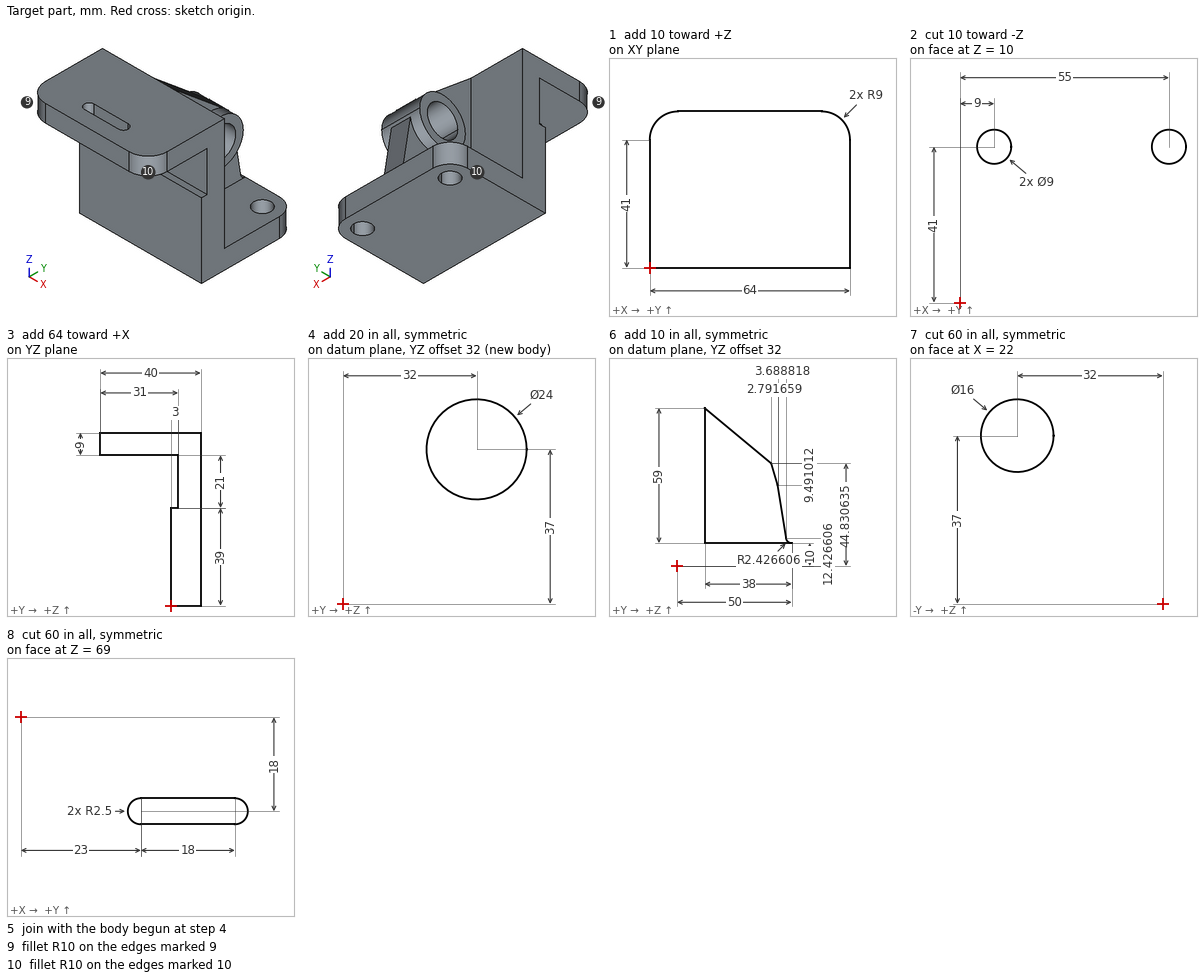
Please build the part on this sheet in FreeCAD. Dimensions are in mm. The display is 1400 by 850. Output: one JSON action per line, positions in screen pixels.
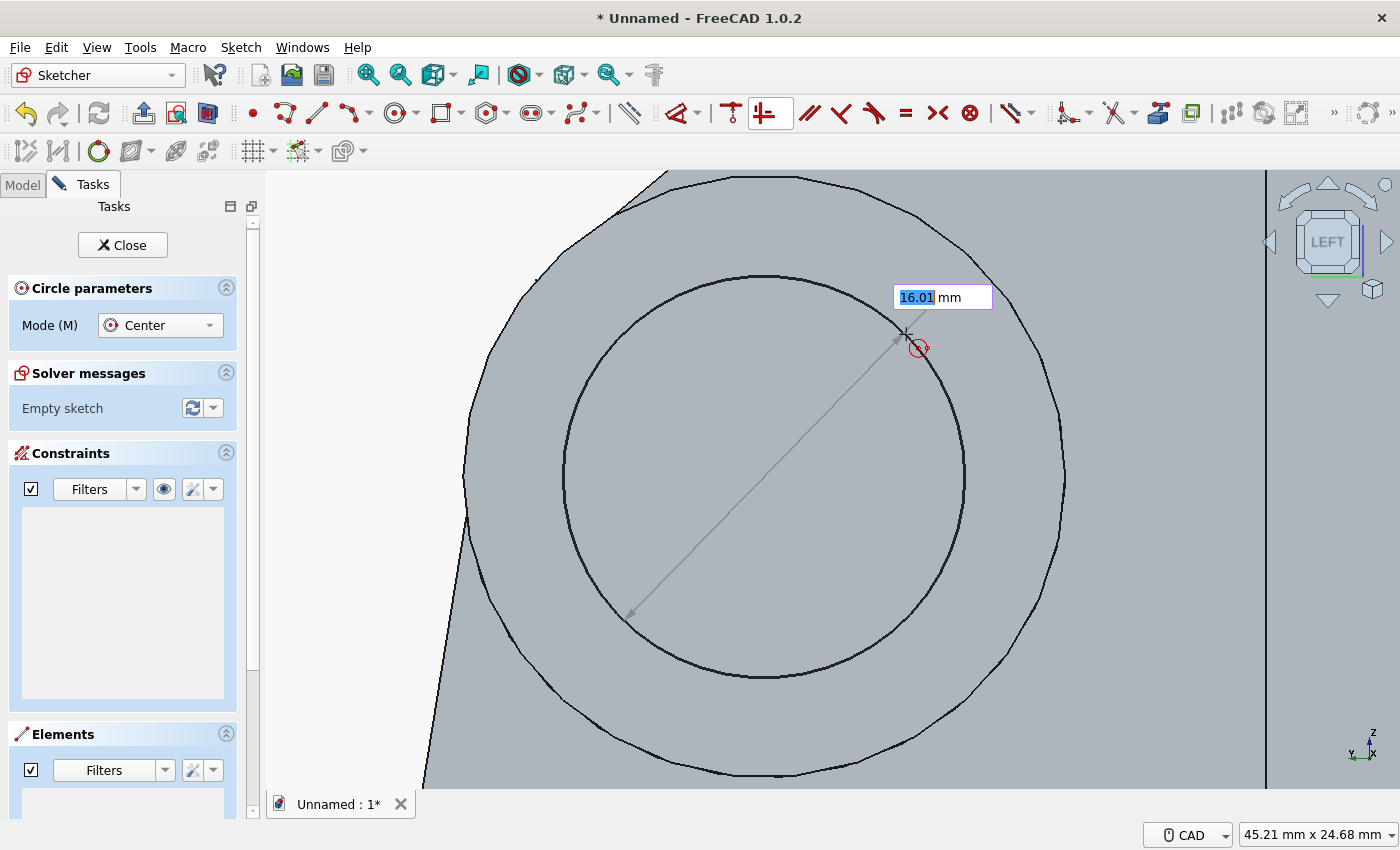
{"action": "type", "text": "16"}
{"action": "key", "text": "Return"}
{"action": "key", "text": "Escape"}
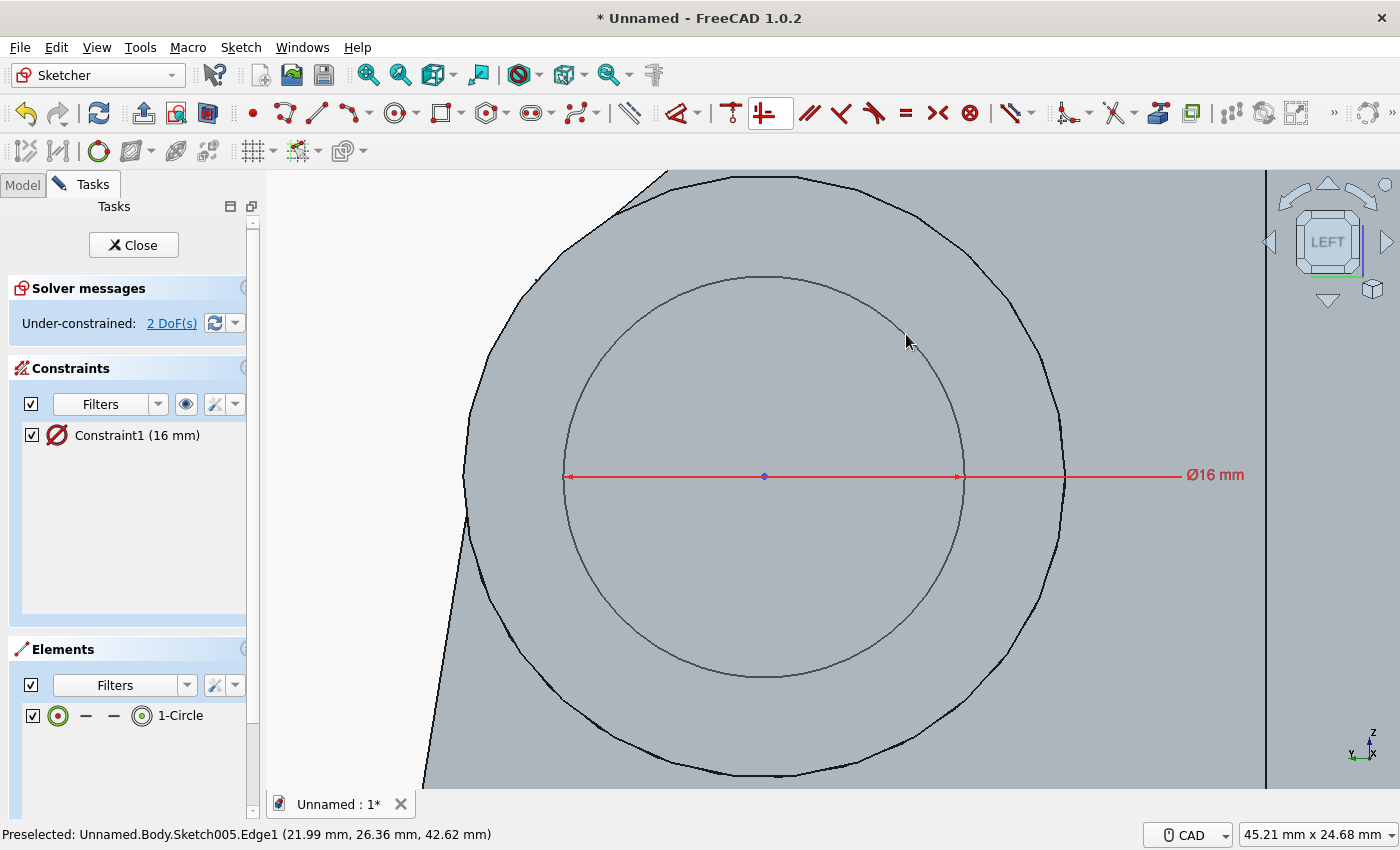
{"action": "left_click", "coordinate": [676, 114]}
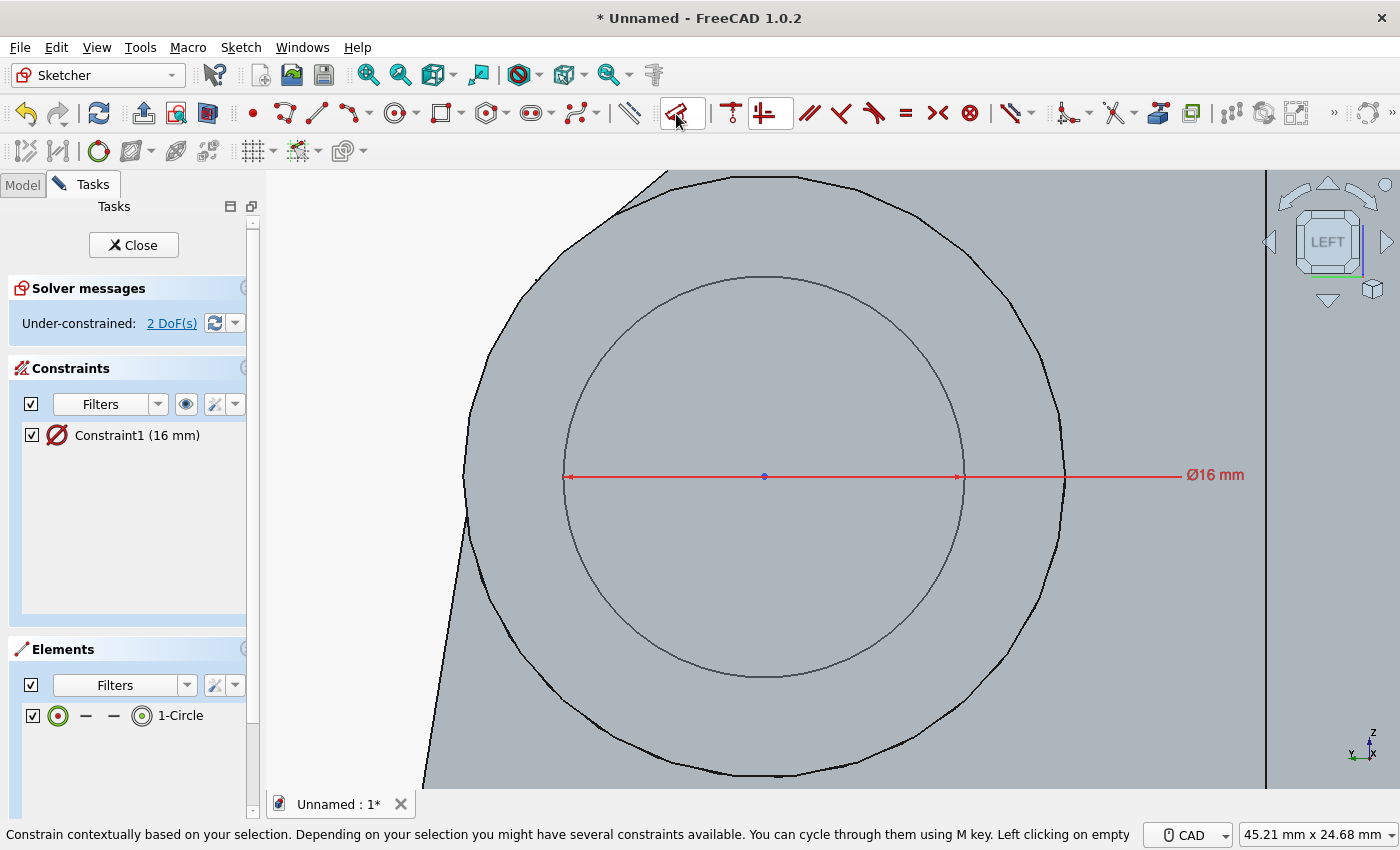
{"action": "left_click", "coordinate": [764, 477]}
{"action": "left_click", "coordinate": [999, 443]}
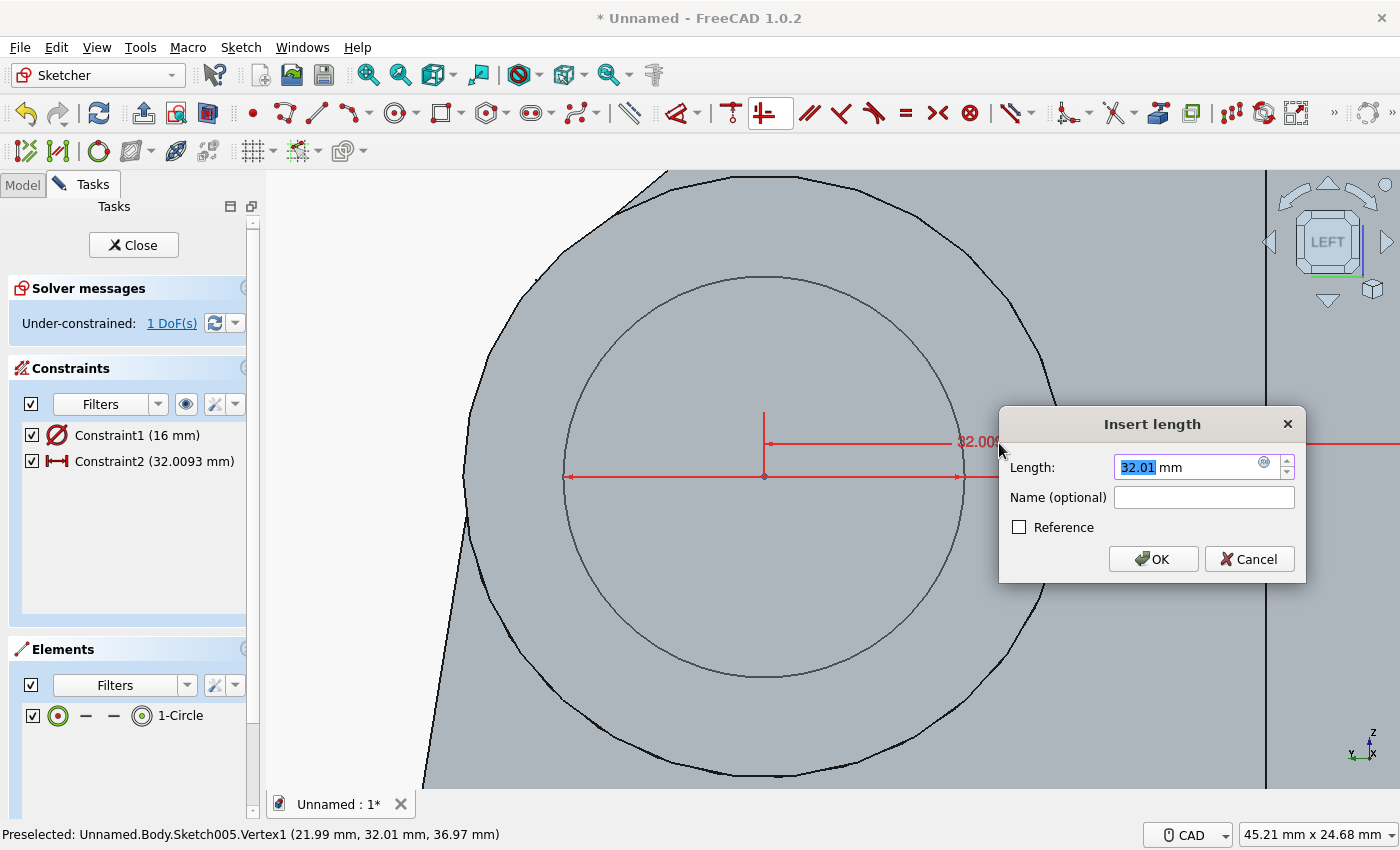
{"action": "type", "text": "32"}
{"action": "key", "text": "Return"}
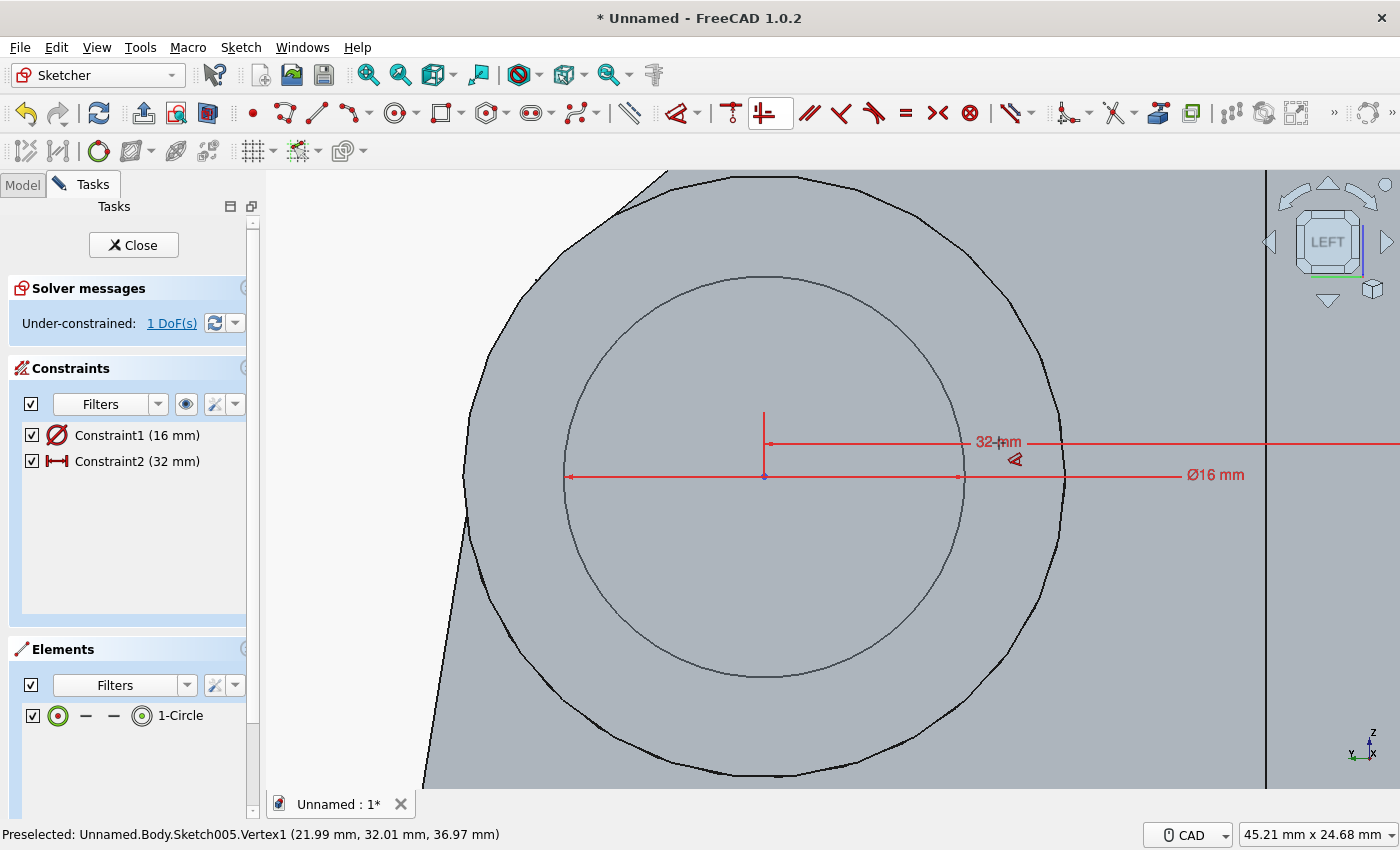
{"action": "left_click", "coordinate": [764, 477]}
{"action": "left_click", "coordinate": [730, 619]}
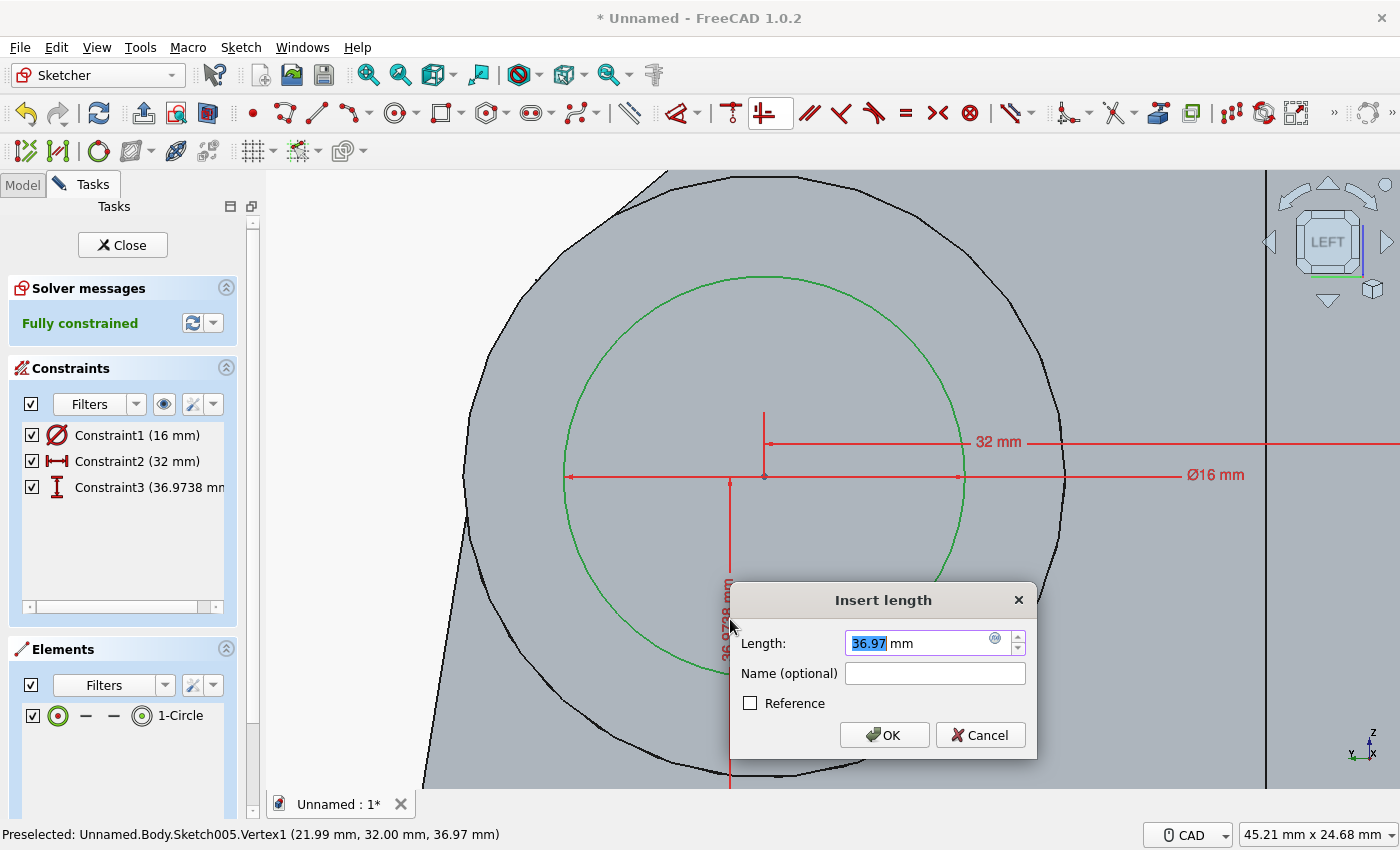
{"action": "type", "text": "37"}
{"action": "key", "text": "Return"}
{"action": "key", "text": "Escape"}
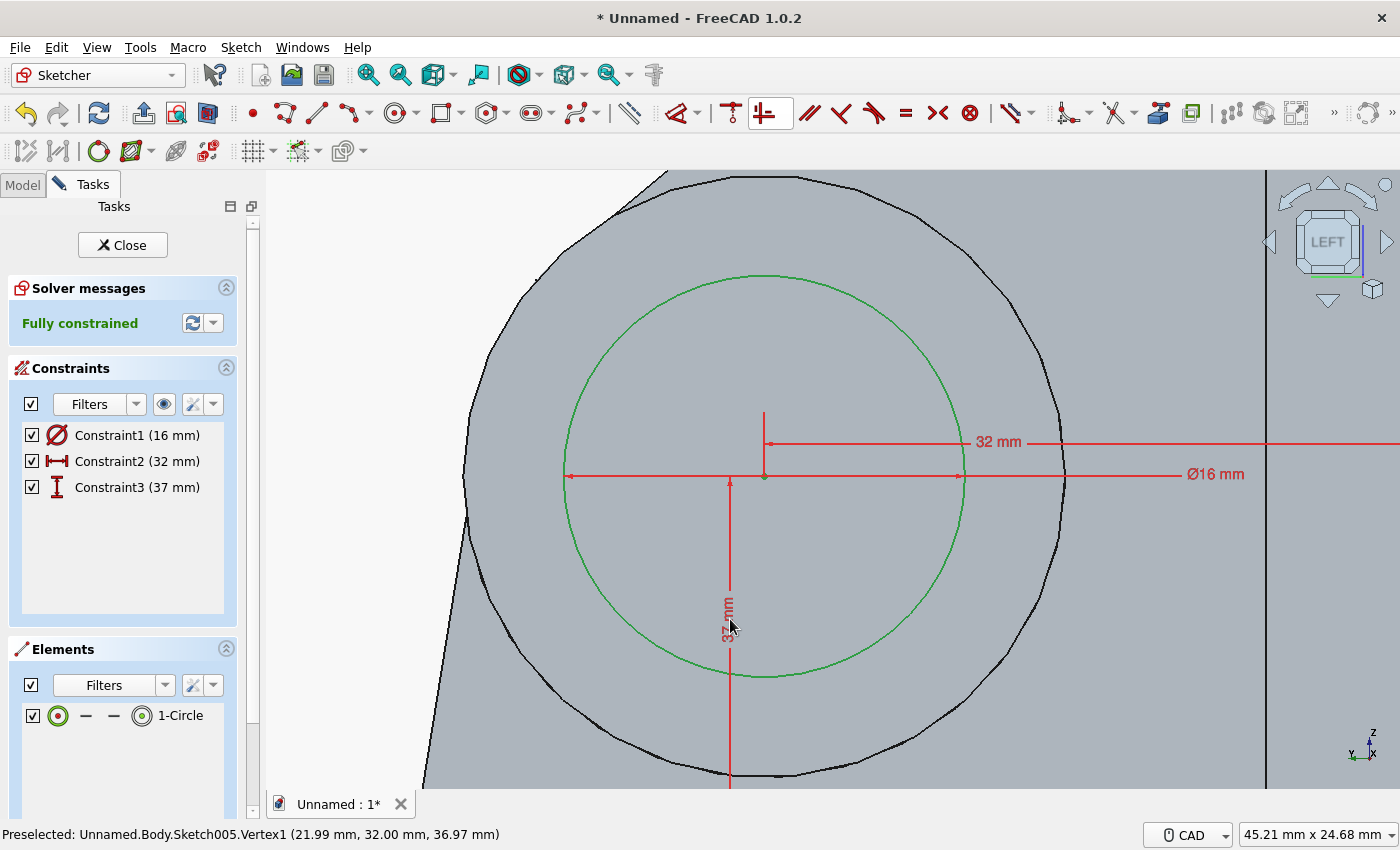
{"action": "left_click", "coordinate": [123, 245]}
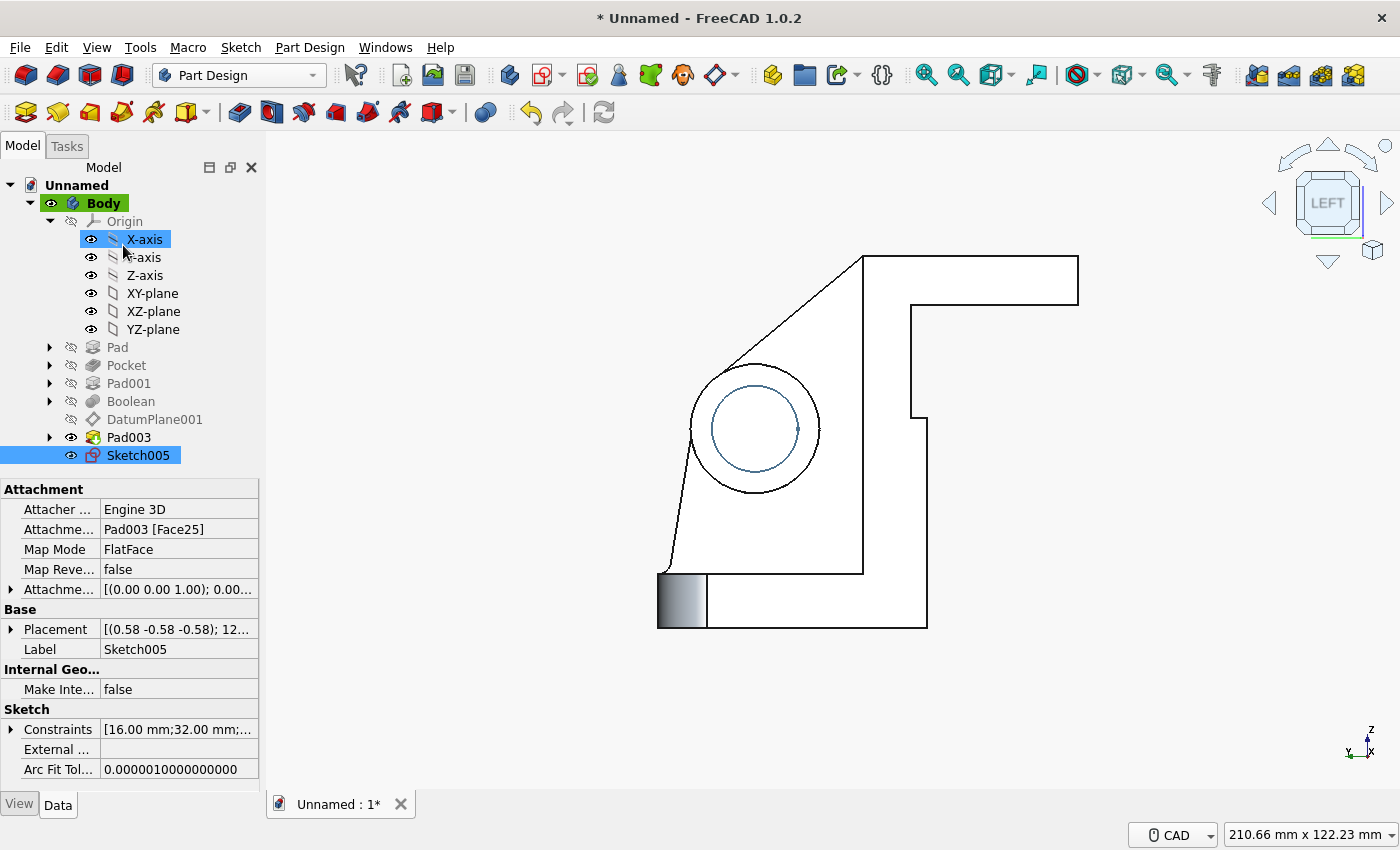
{"action": "left_click", "coordinate": [240, 112]}